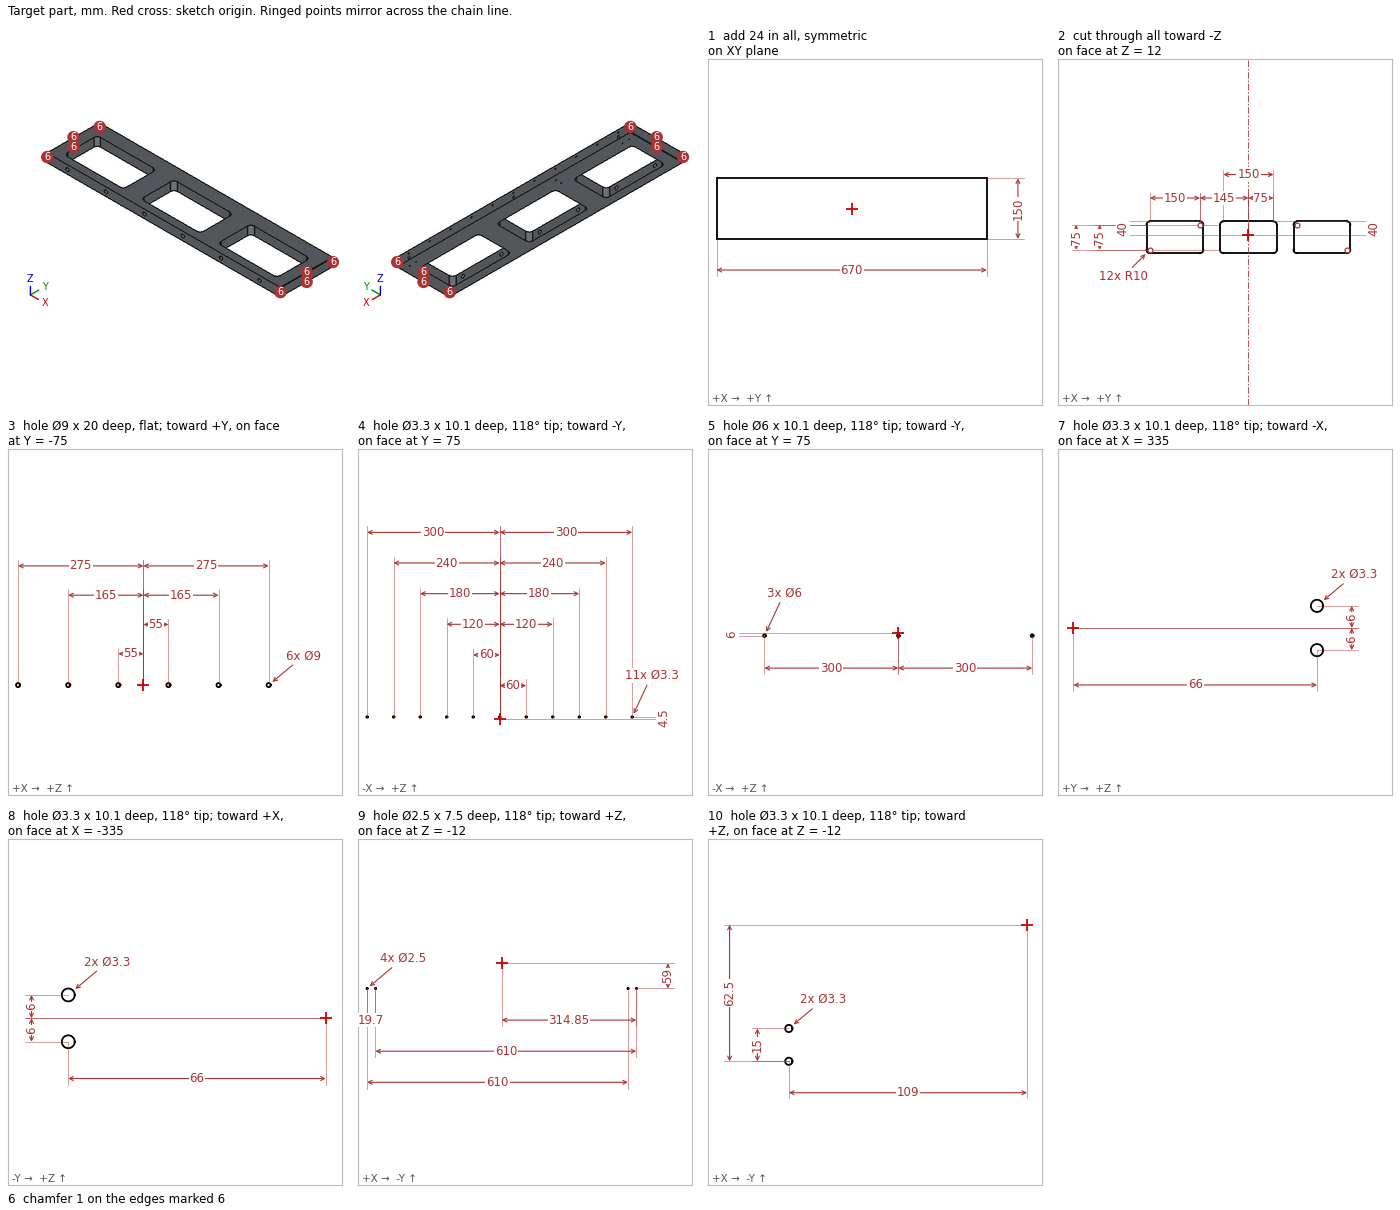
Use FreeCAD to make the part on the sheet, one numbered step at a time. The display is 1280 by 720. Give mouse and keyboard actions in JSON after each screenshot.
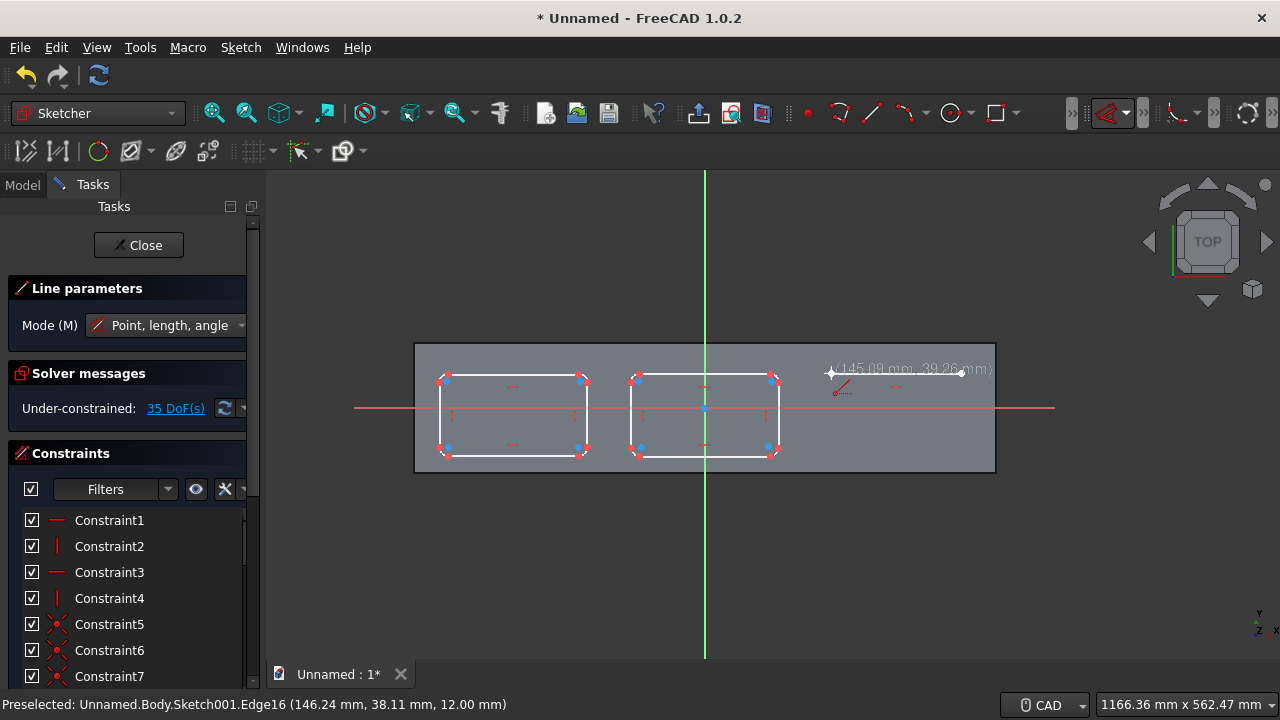
{"action": "scroll", "coordinate": [822, 382], "scroll_direction": "up", "scroll_amount": 2}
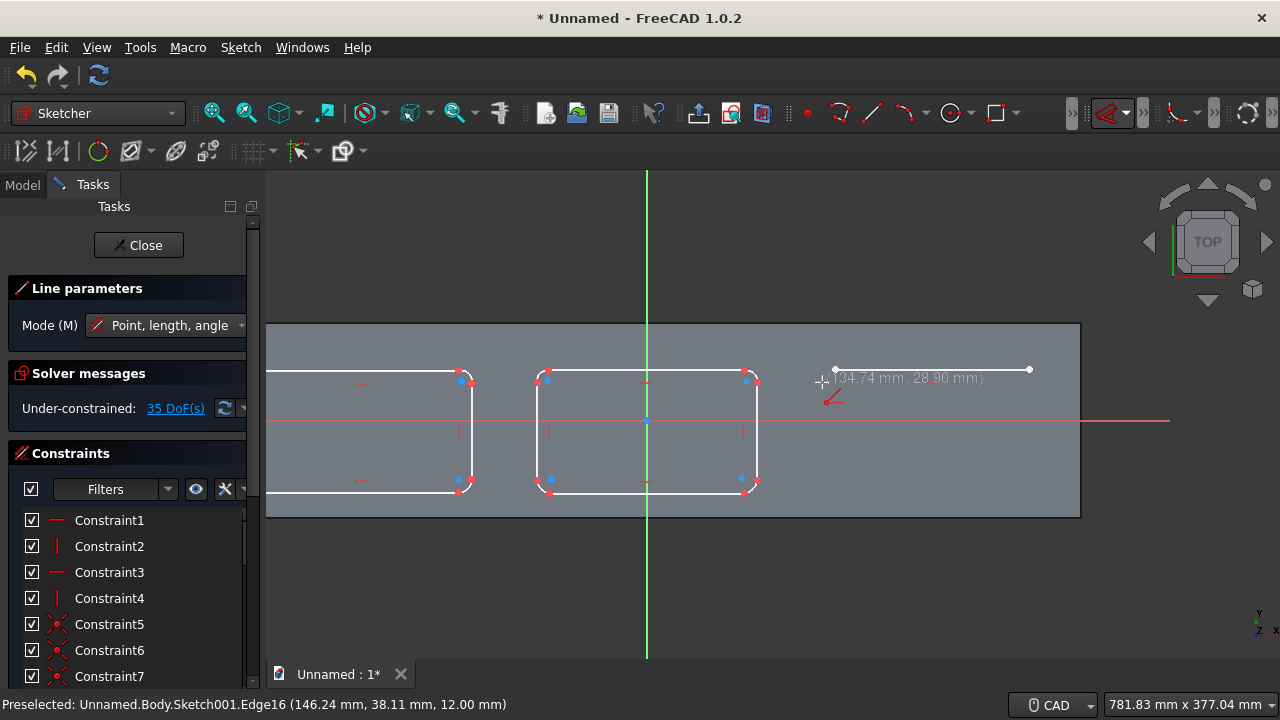
{"action": "left_click", "coordinate": [822, 382]}
{"action": "left_click", "coordinate": [822, 479]}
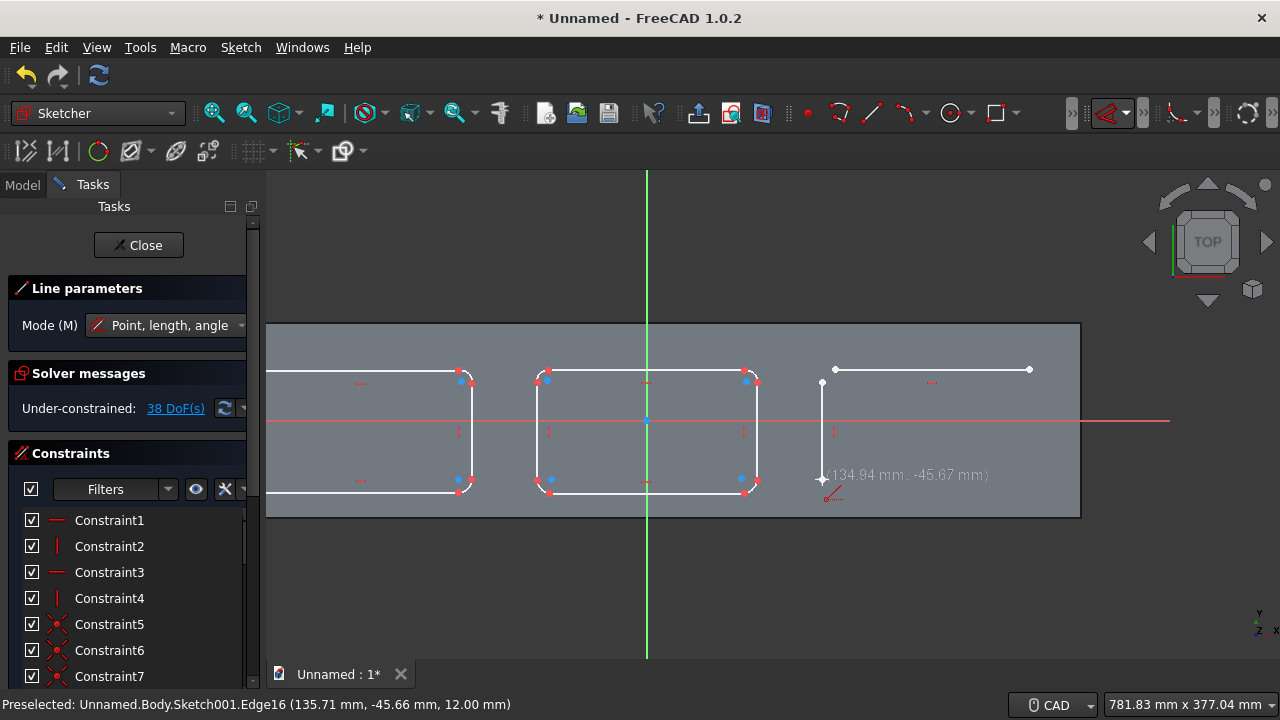
{"action": "left_click", "coordinate": [835, 492]}
{"action": "left_click", "coordinate": [1030, 492]}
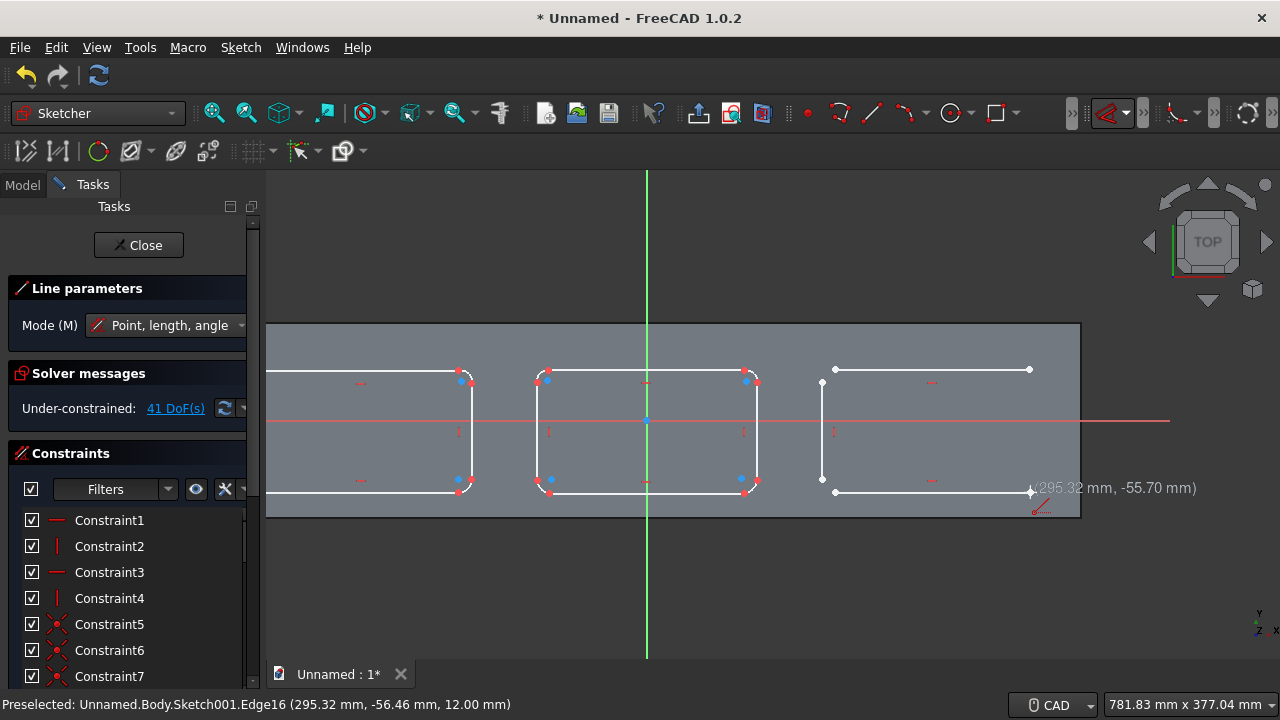
{"action": "left_click", "coordinate": [1043, 479]}
{"action": "left_click", "coordinate": [1043, 382]}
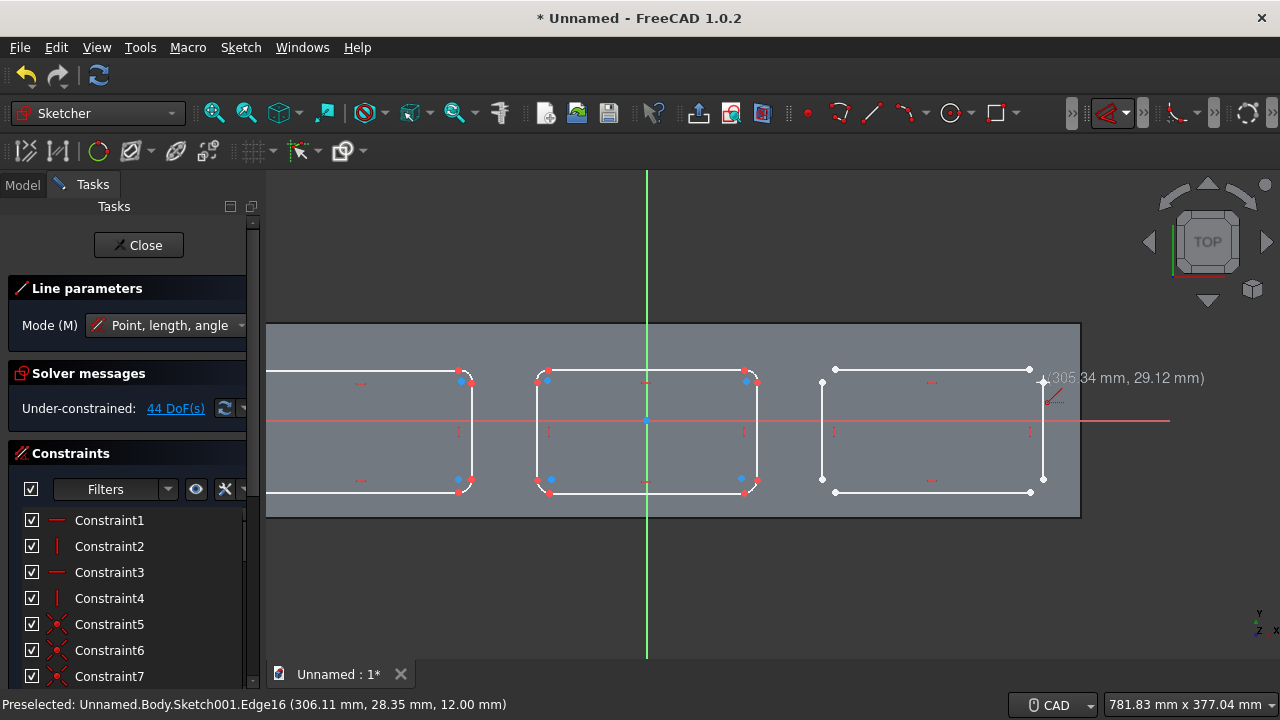
{"action": "left_click", "coordinate": [906, 114]}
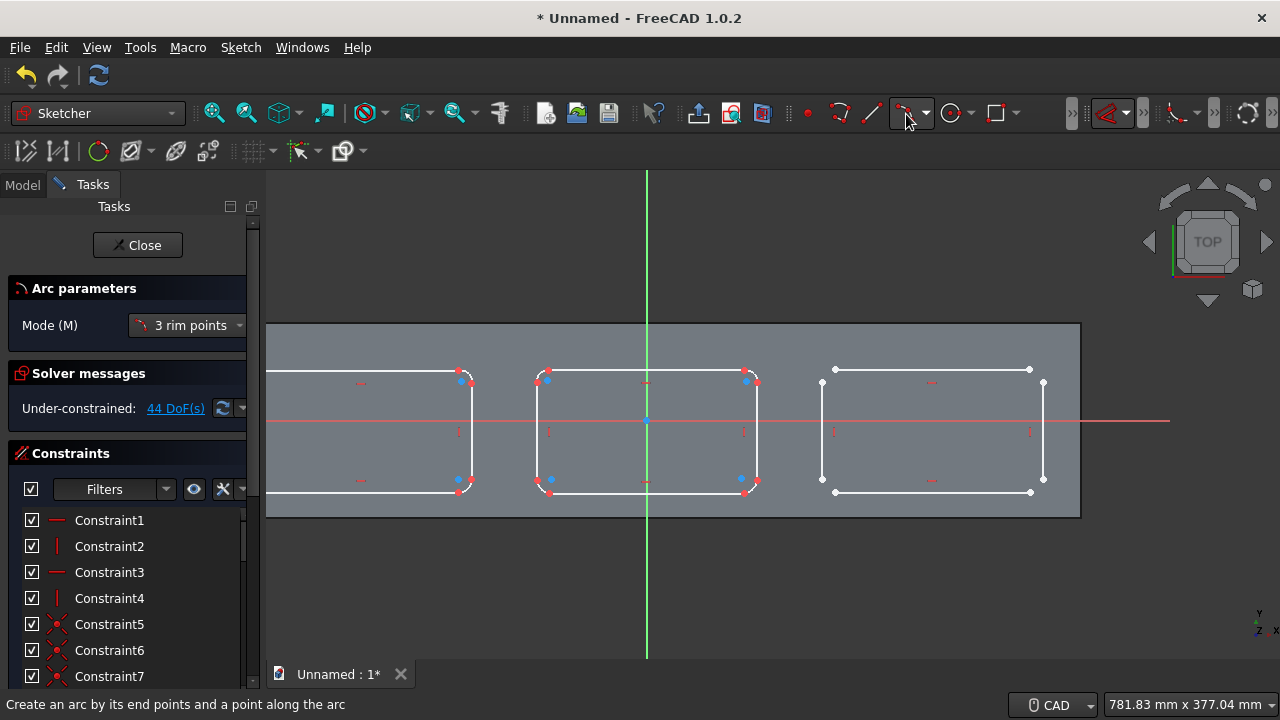
{"action": "left_click", "coordinate": [835, 370]}
{"action": "left_click", "coordinate": [822, 383]}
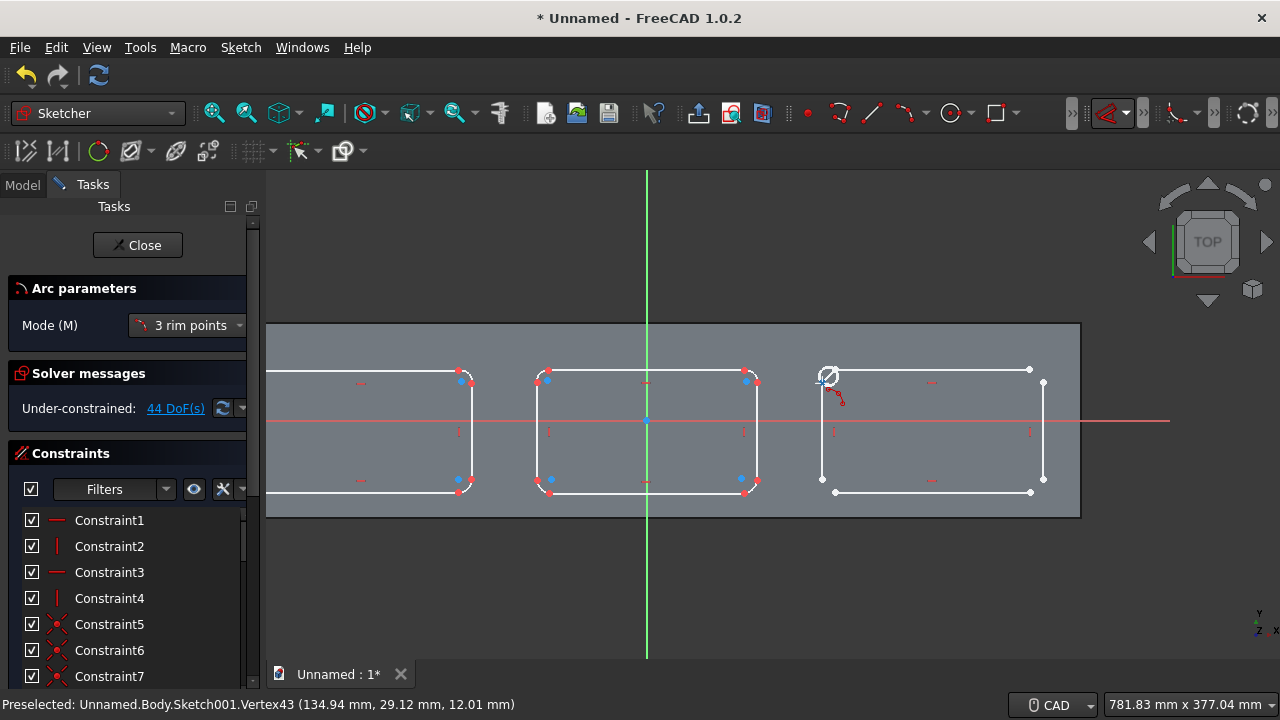
{"action": "scroll", "coordinate": [826, 373], "scroll_direction": "up", "scroll_amount": 8}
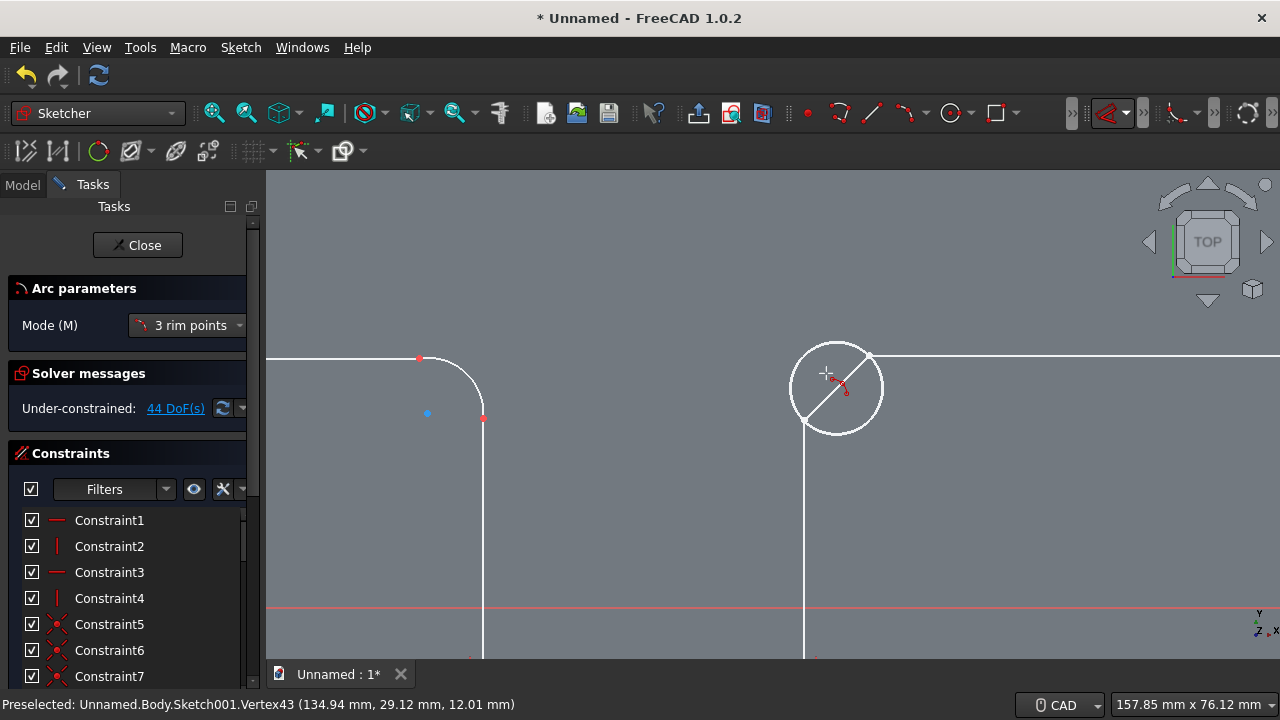
{"action": "left_click", "coordinate": [823, 370]}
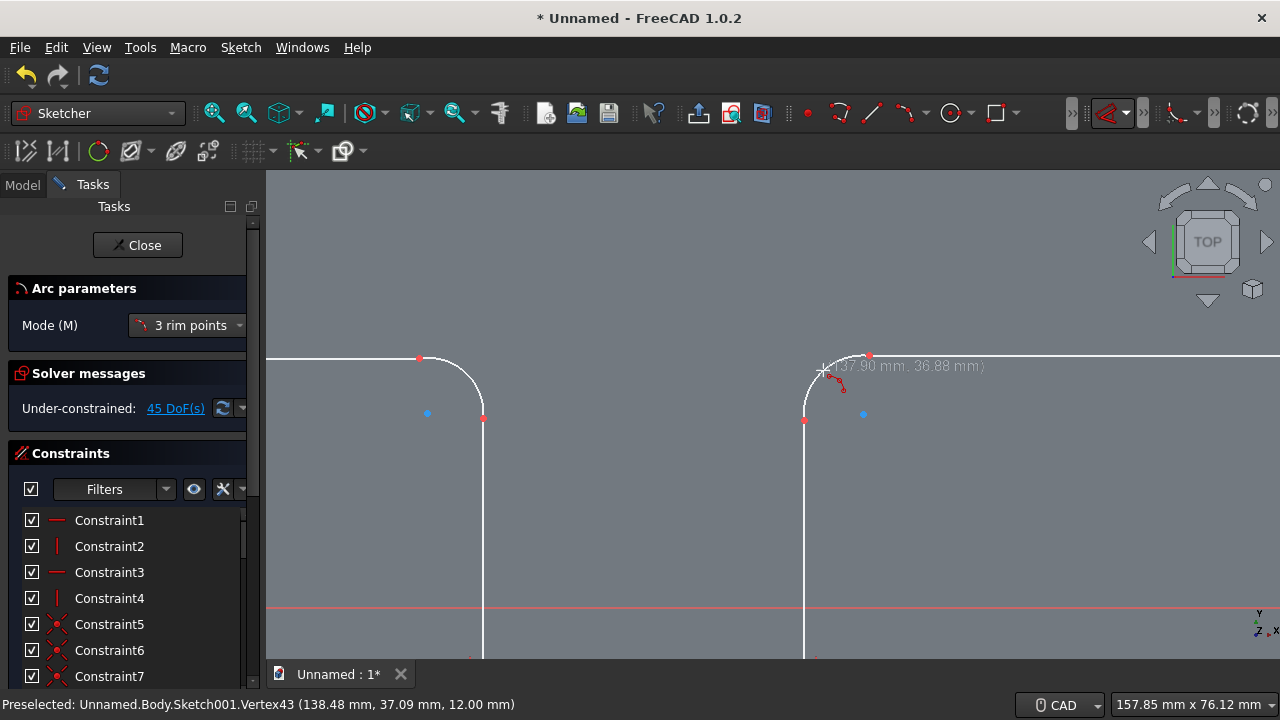
{"action": "scroll", "coordinate": [825, 377], "scroll_direction": "down", "scroll_amount": 10}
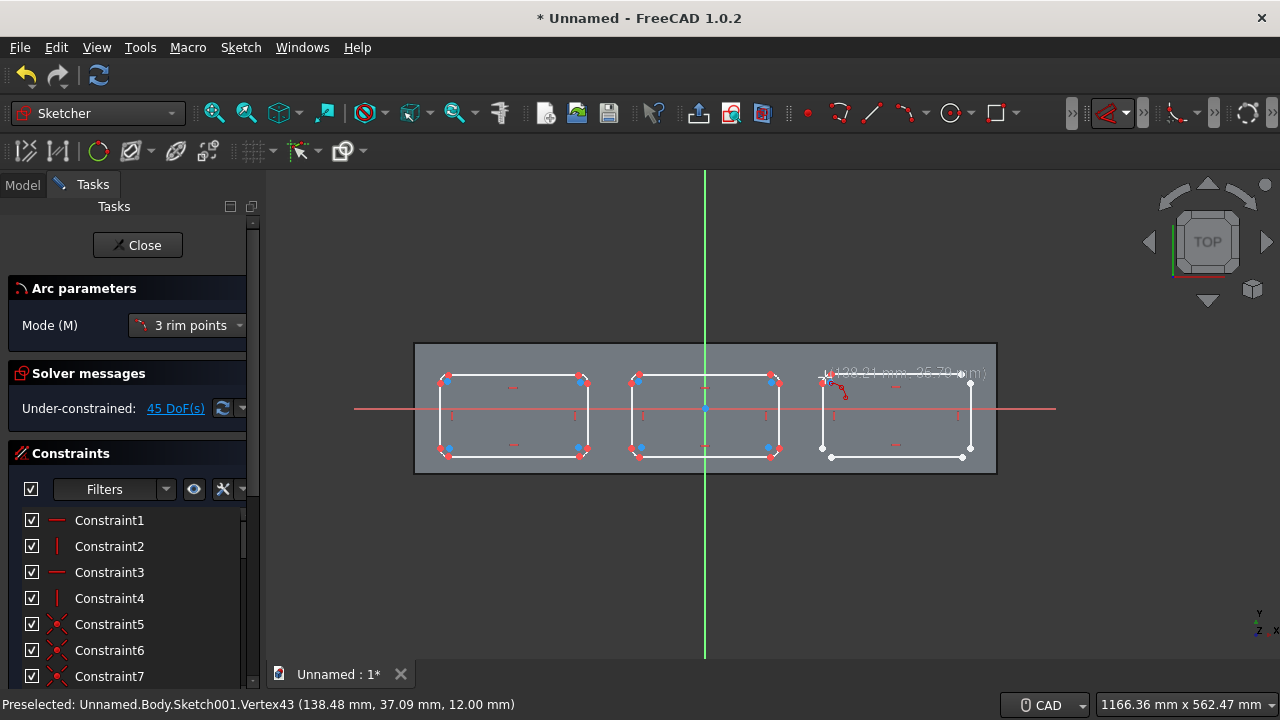
{"action": "scroll", "coordinate": [823, 448], "scroll_direction": "up", "scroll_amount": 2}